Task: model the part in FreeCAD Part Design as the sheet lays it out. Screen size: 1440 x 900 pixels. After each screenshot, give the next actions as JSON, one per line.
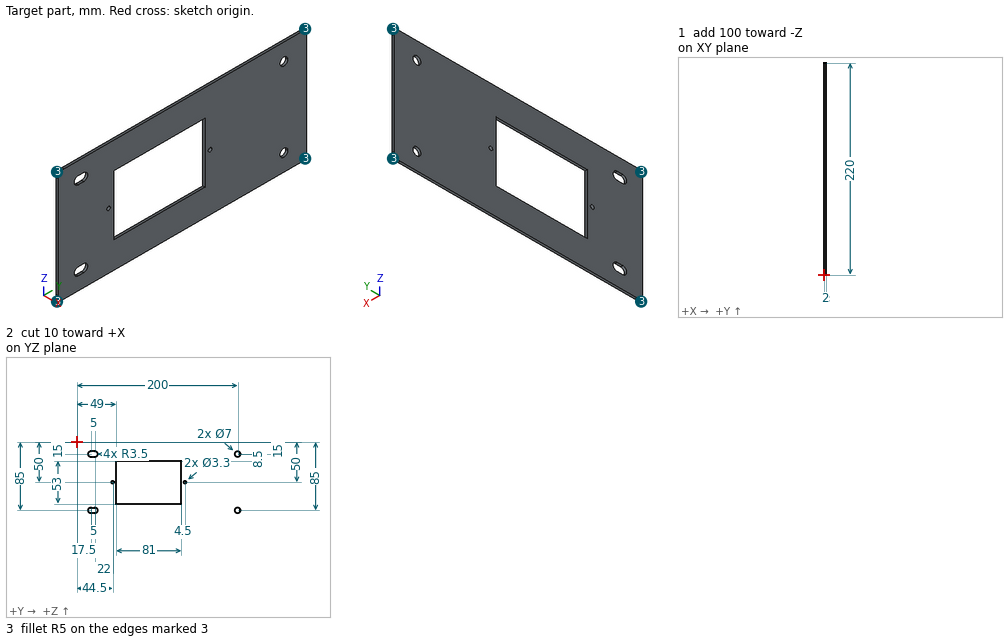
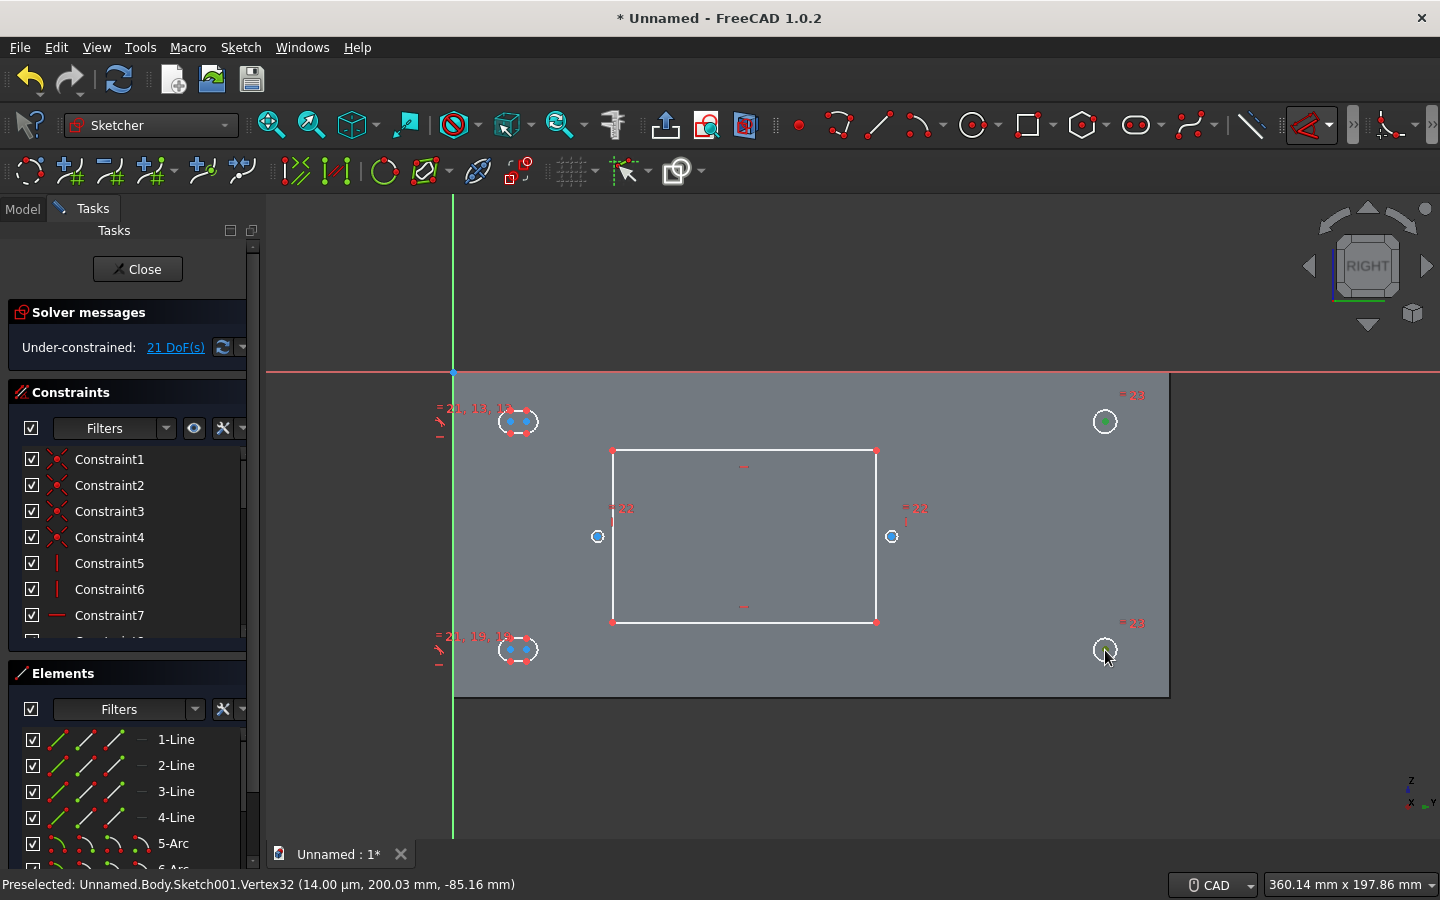
{"action": "key", "text": "v"}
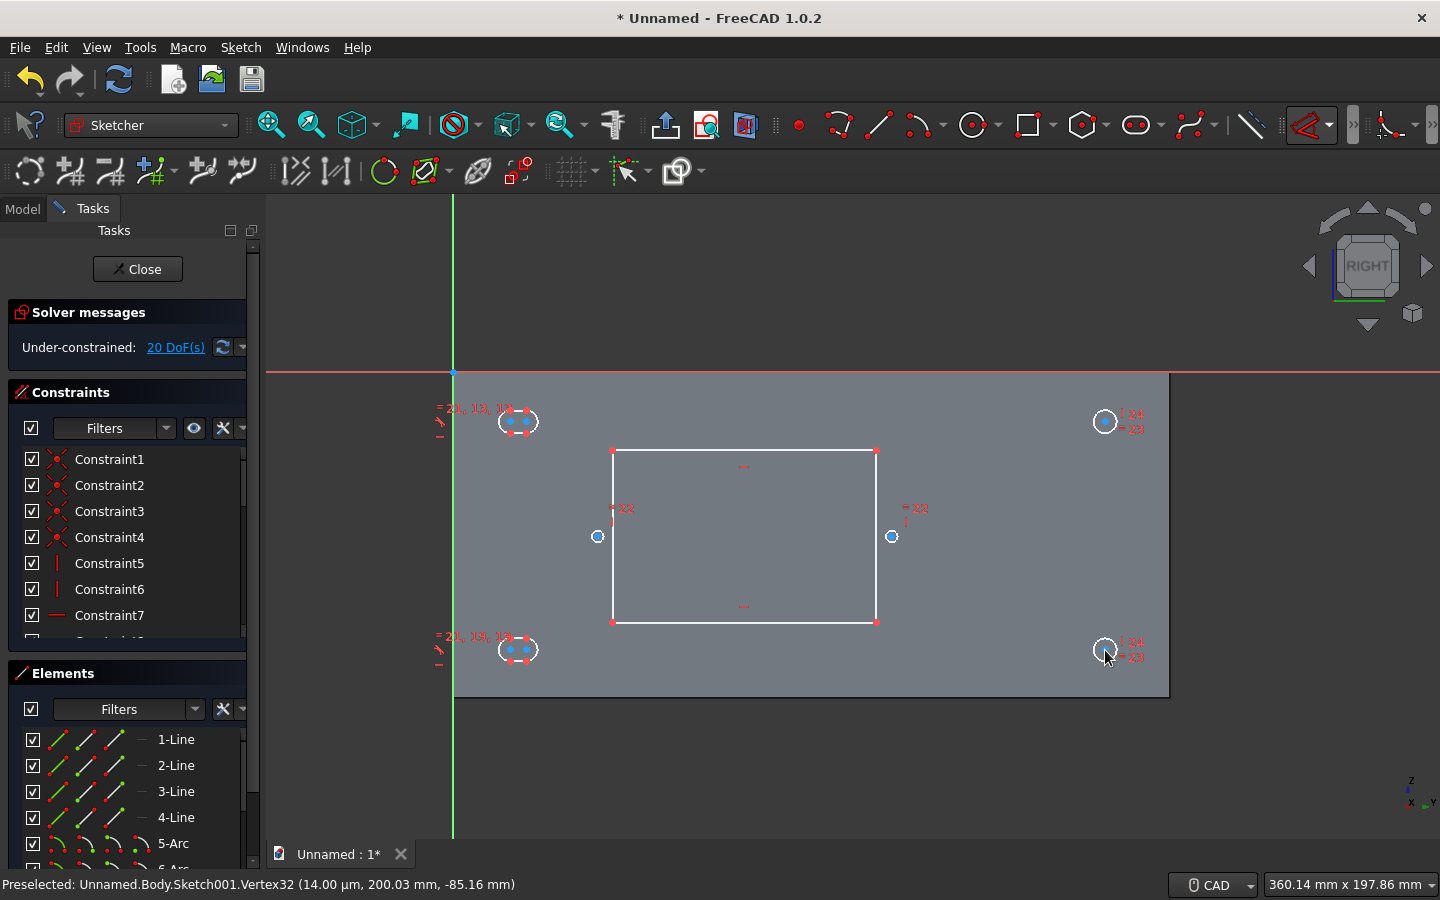
{"action": "scroll", "coordinate": [501, 415], "scroll_direction": "up", "scroll_amount": 7}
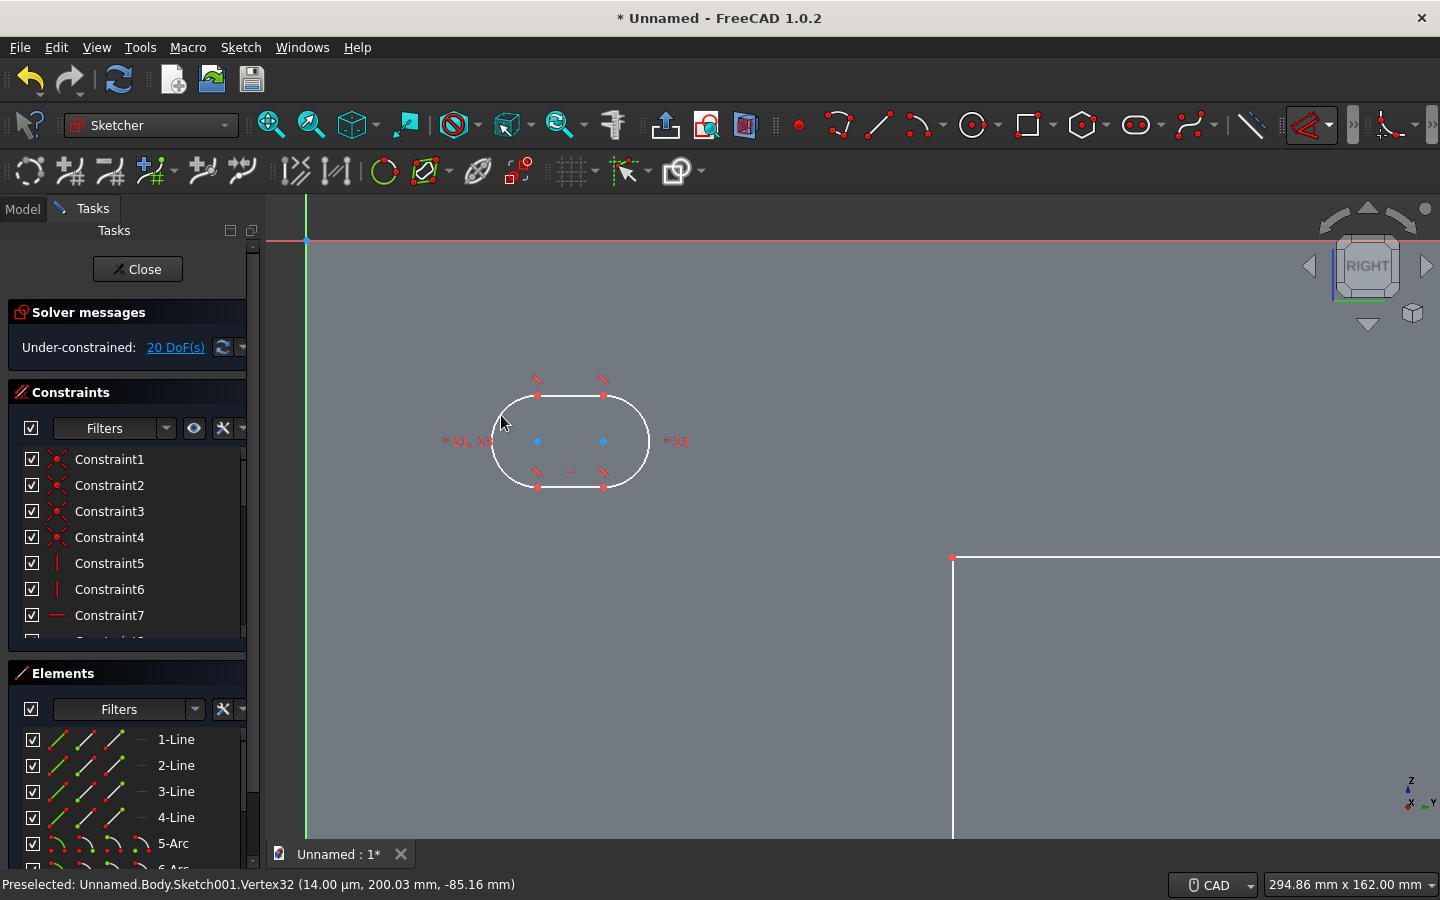
{"action": "left_click", "coordinate": [501, 415]}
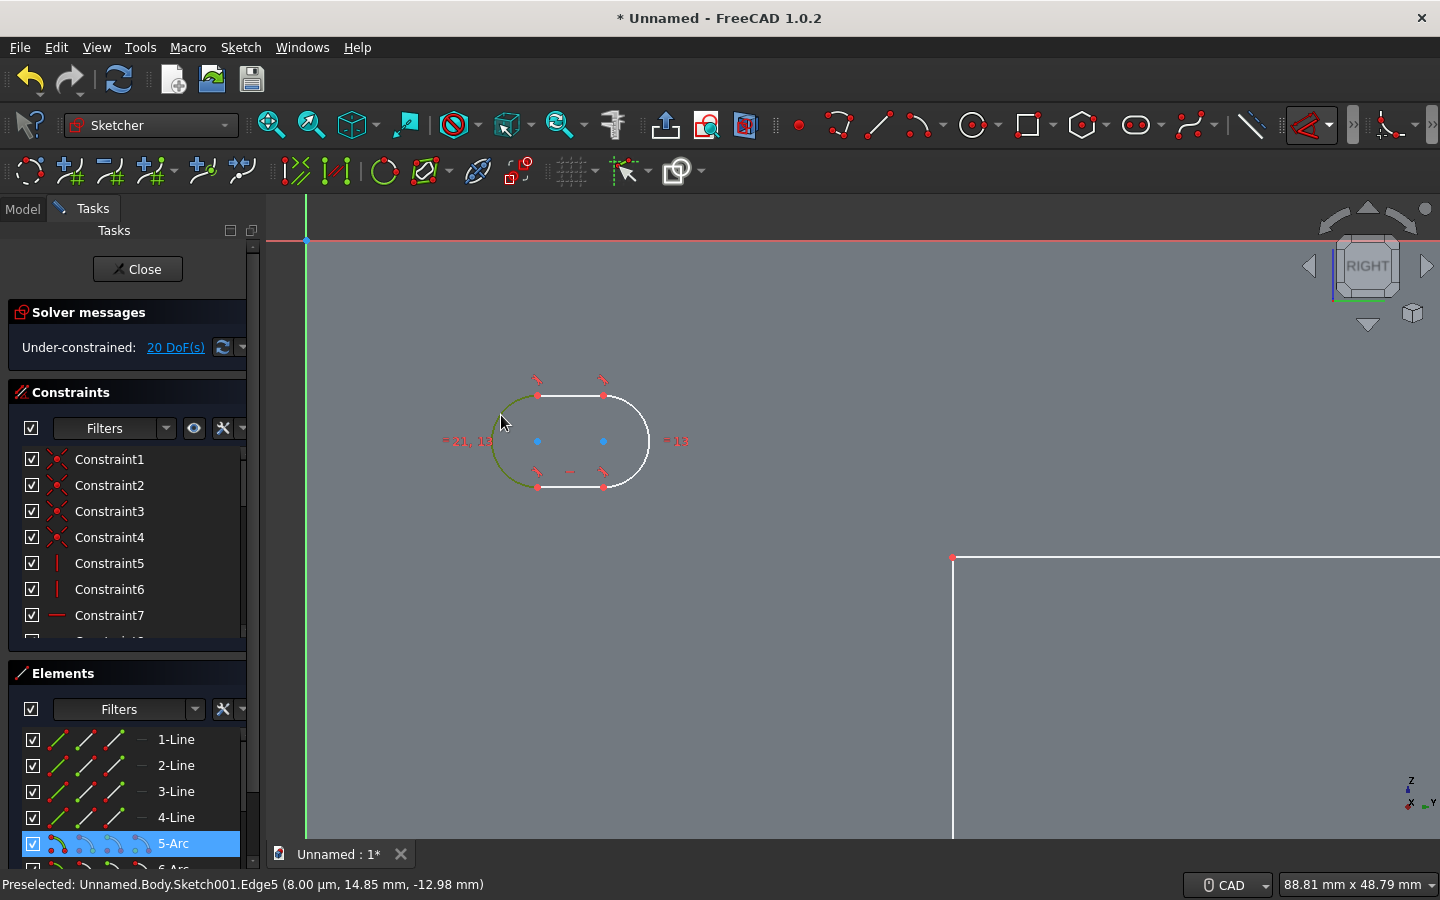
{"action": "key", "text": "k r"}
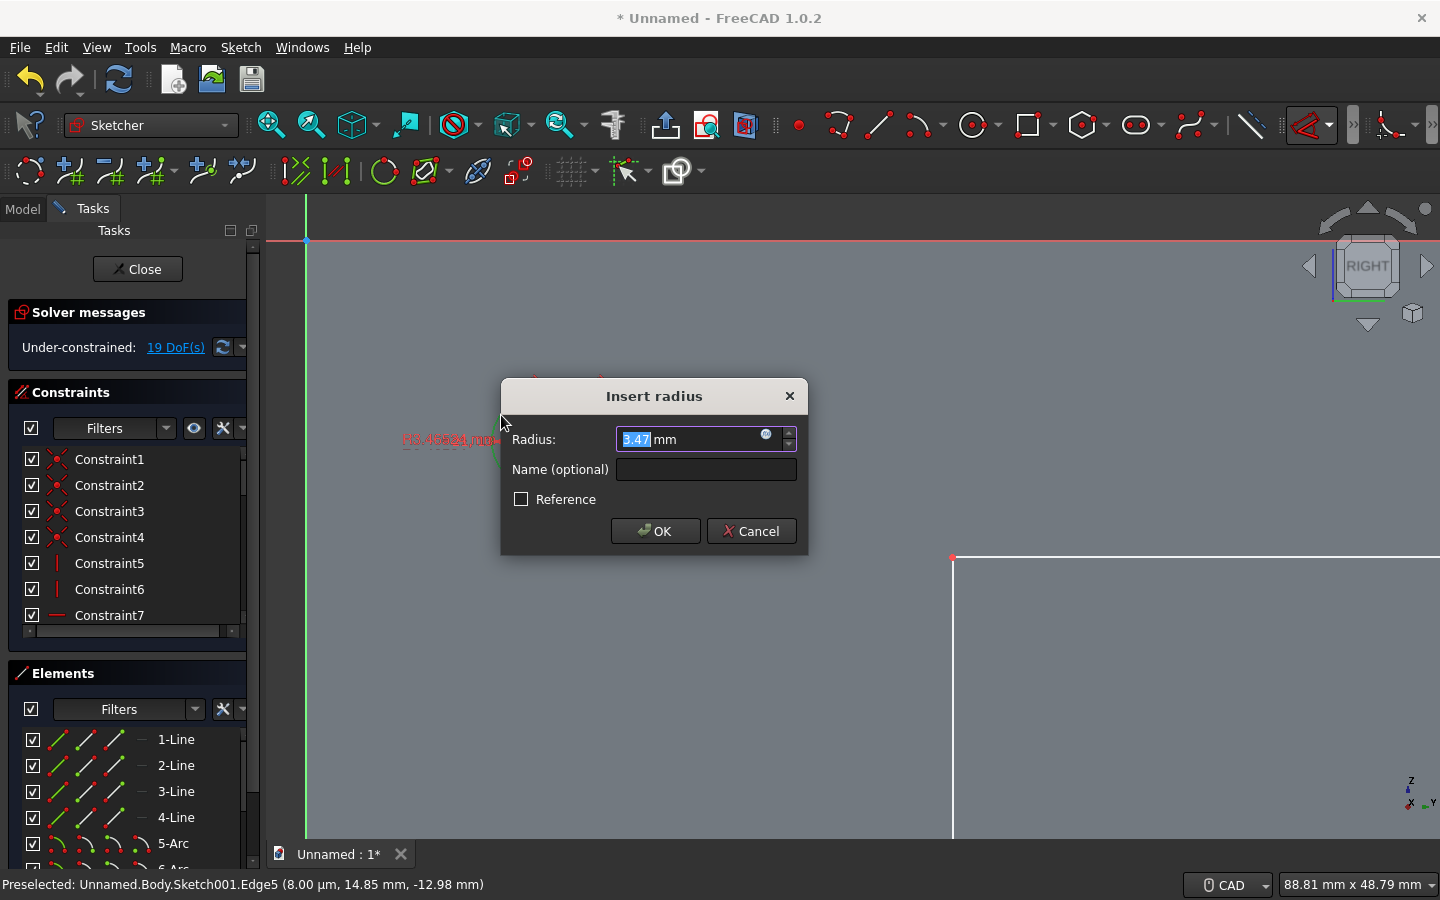
{"action": "type", "text": "3.5"}
{"action": "key", "text": "Return"}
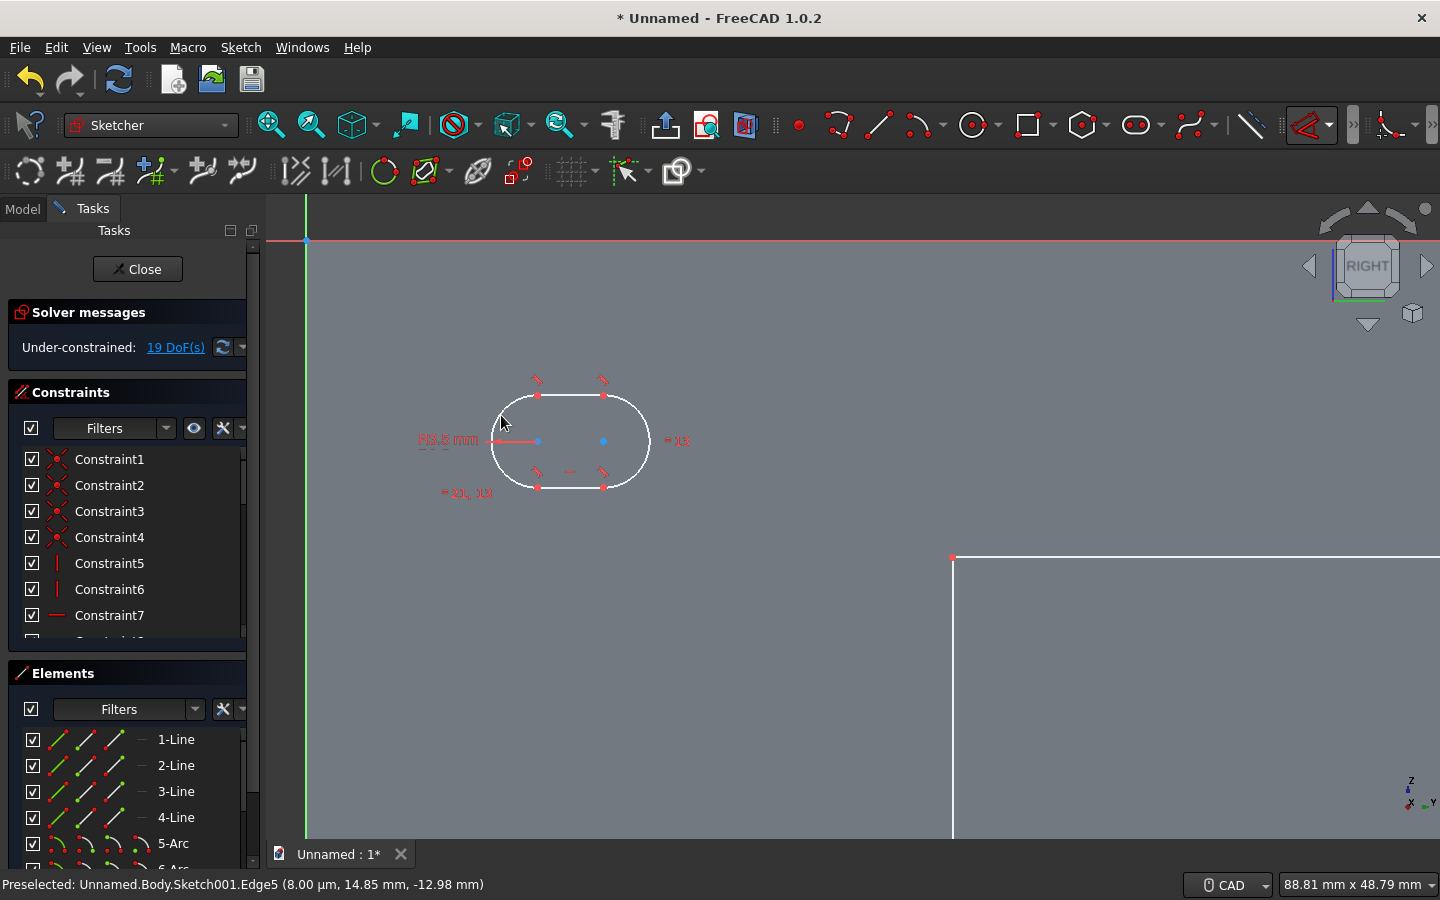
{"action": "scroll", "coordinate": [501, 415], "scroll_direction": "down", "scroll_amount": 7}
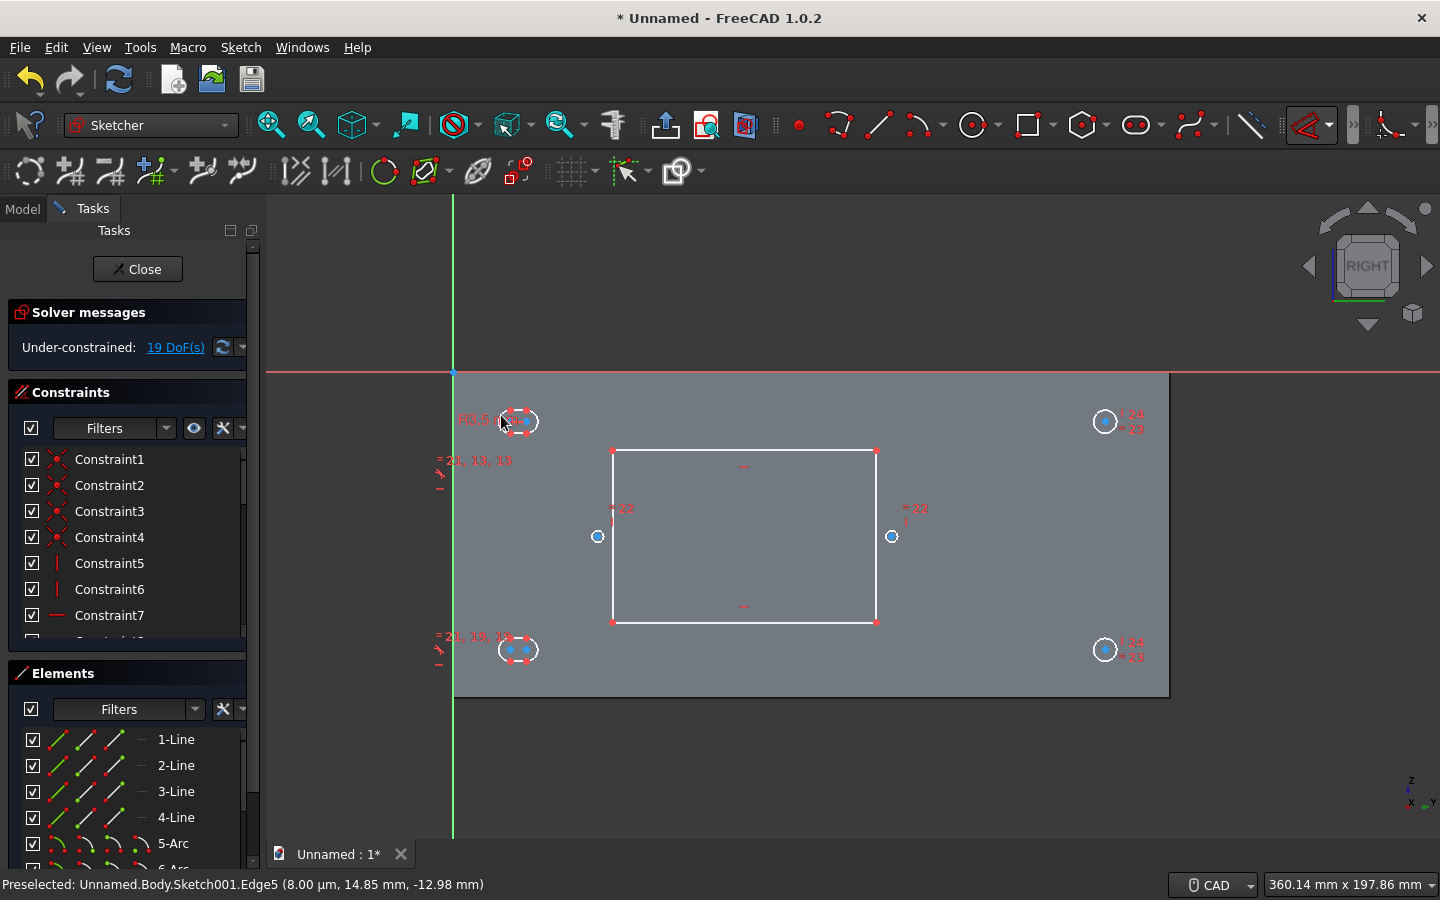
{"action": "scroll", "coordinate": [602, 532], "scroll_direction": "up", "scroll_amount": 7}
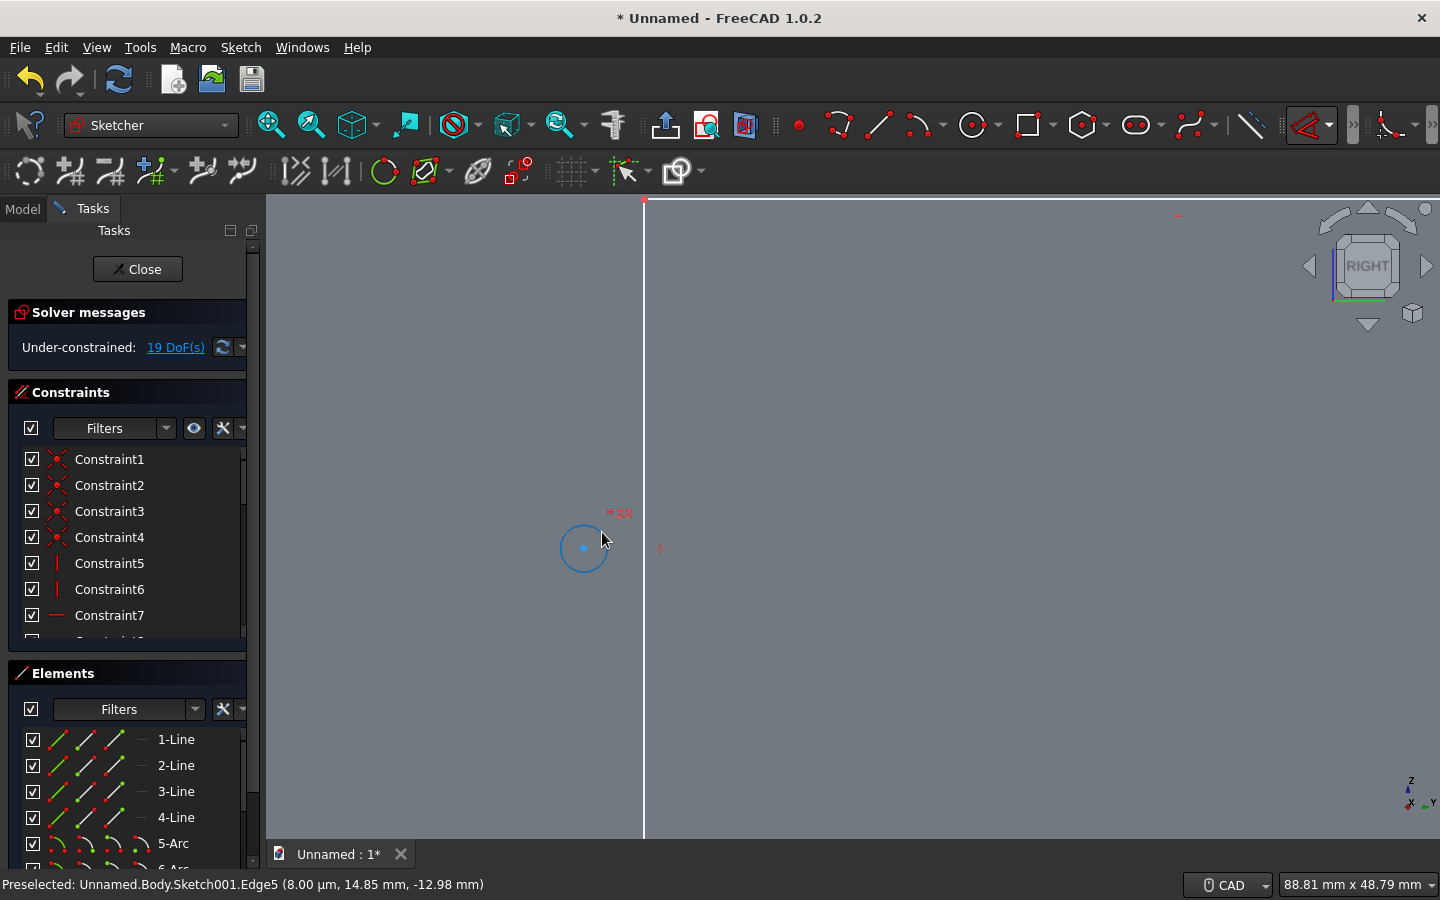
{"action": "left_click", "coordinate": [600, 532]}